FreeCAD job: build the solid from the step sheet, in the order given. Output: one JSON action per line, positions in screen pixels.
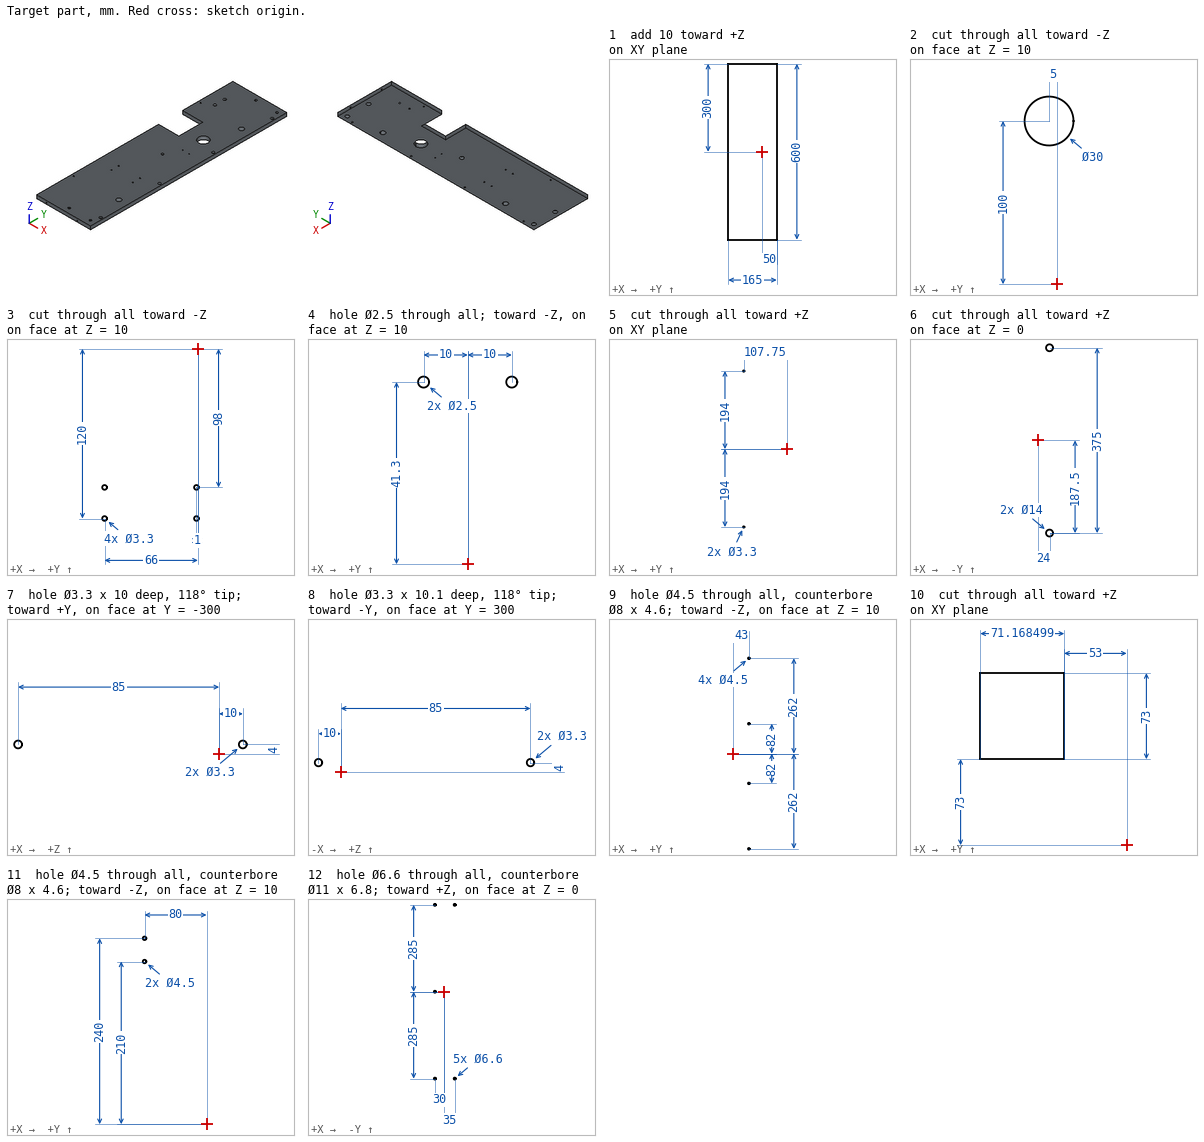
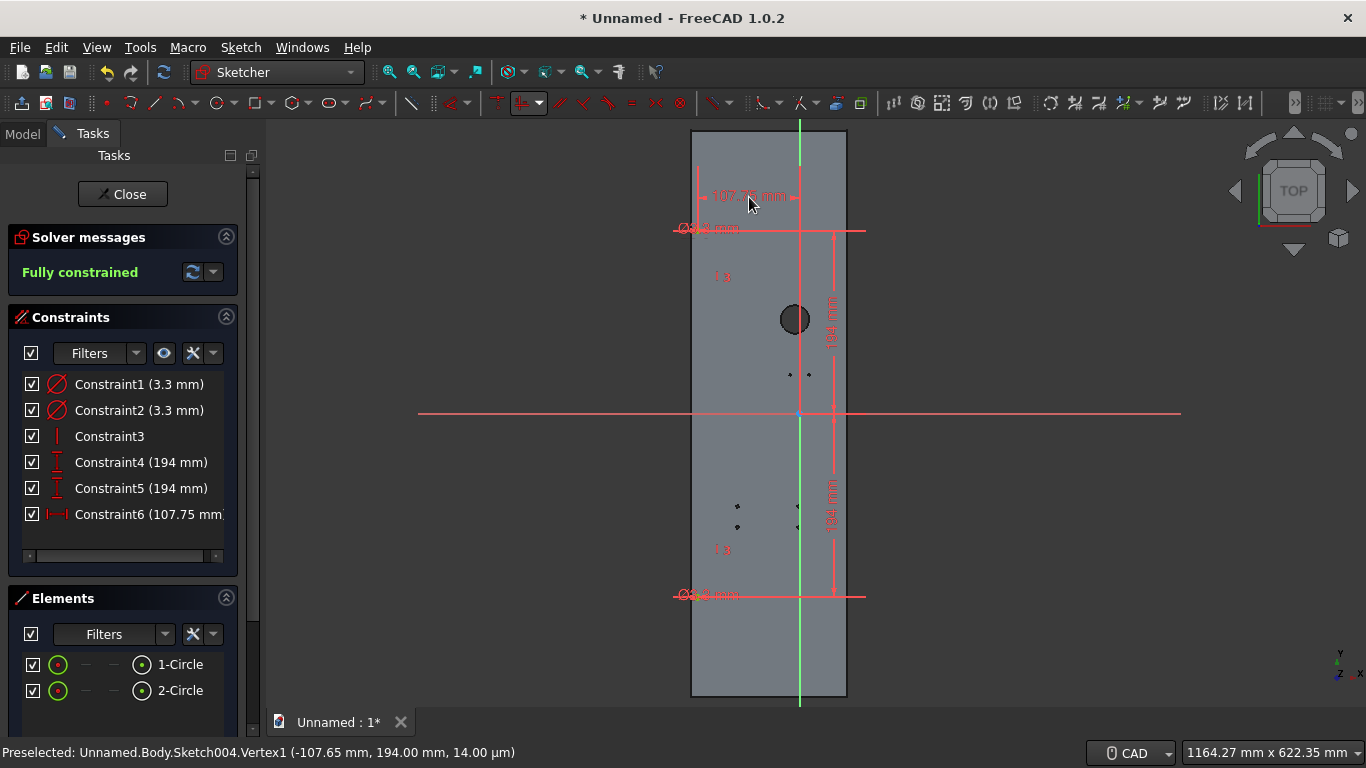
{"action": "left_click", "coordinate": [123, 194]}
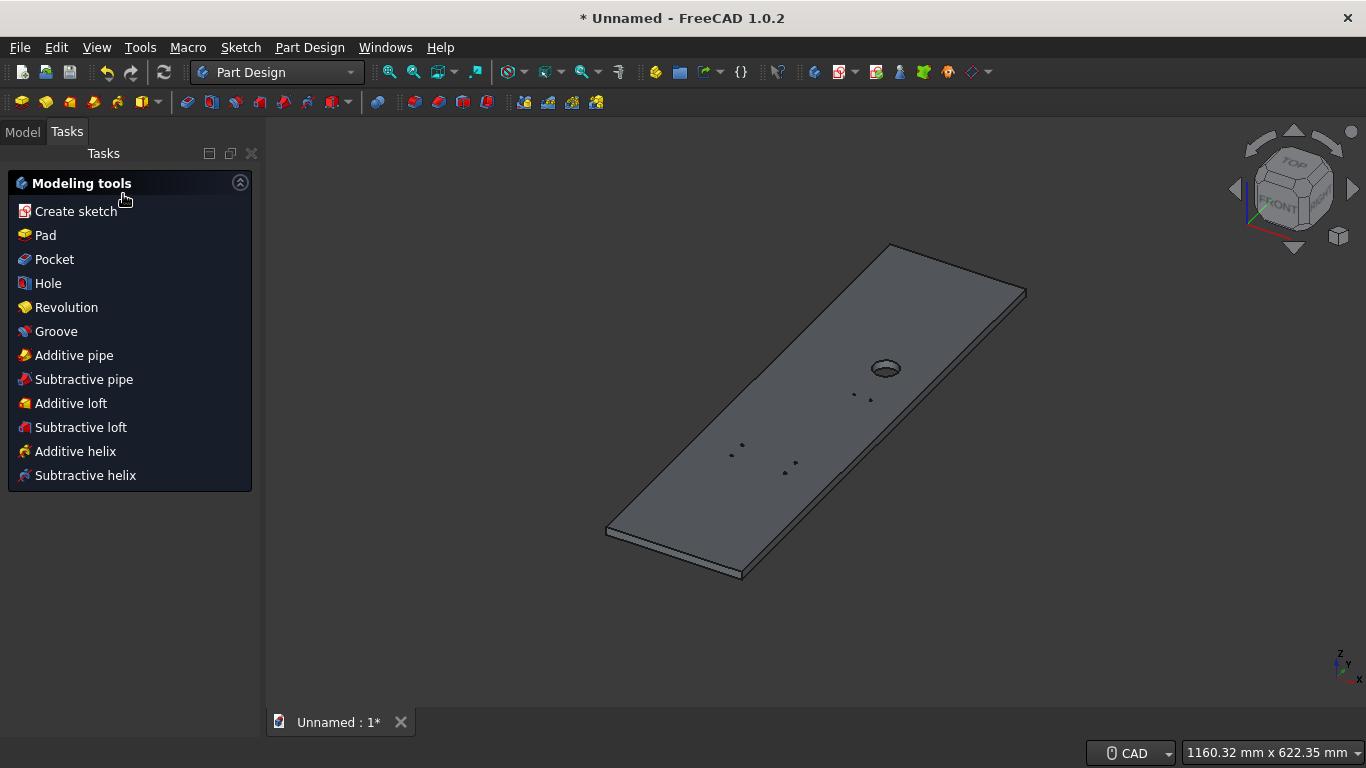
{"action": "left_click", "coordinate": [188, 102]}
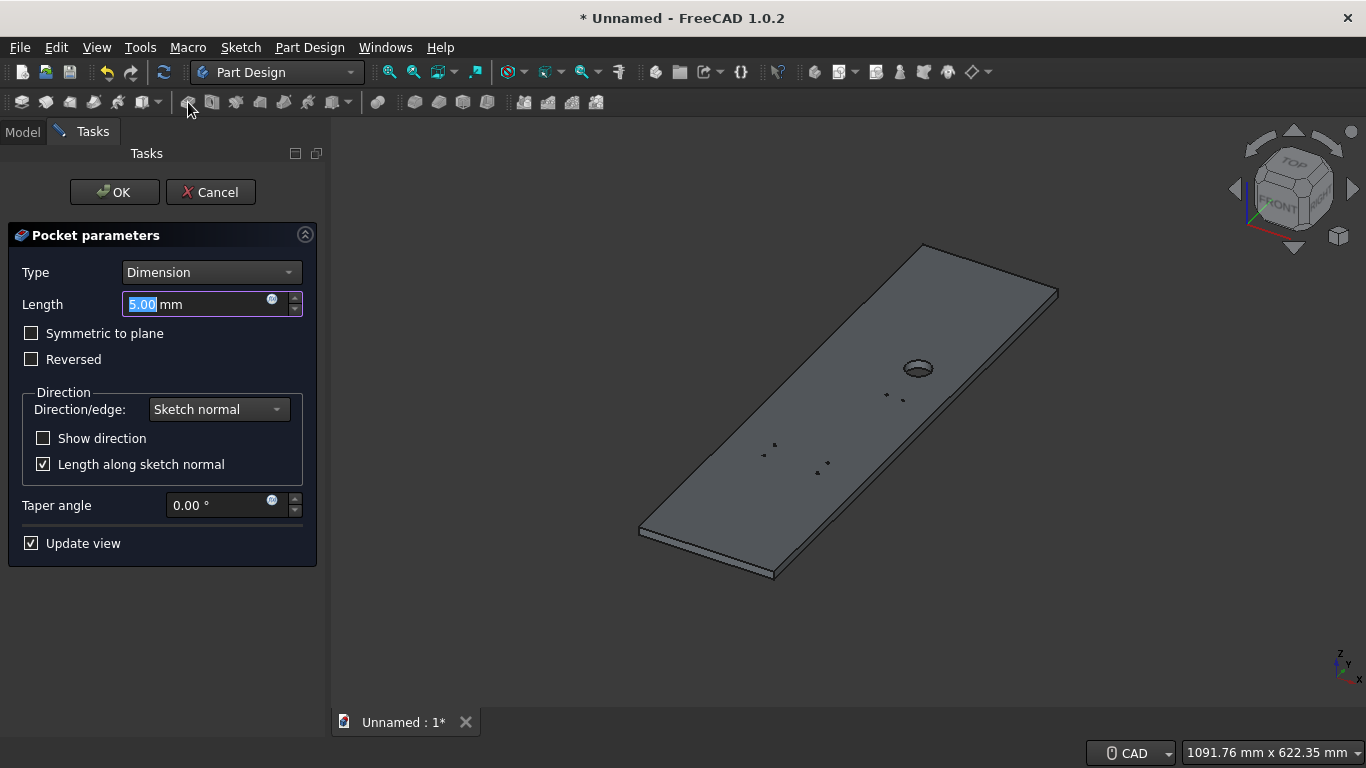
{"action": "left_click", "coordinate": [212, 272]}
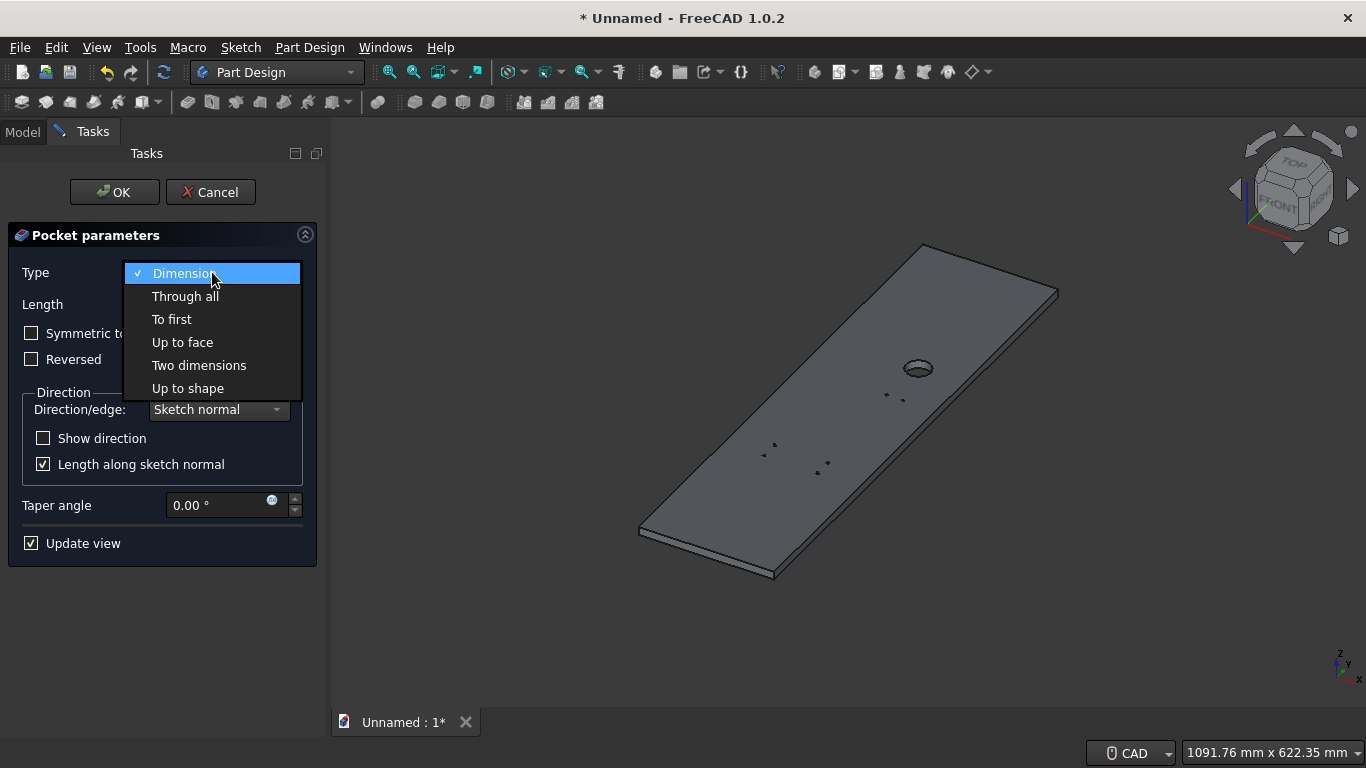
{"action": "left_click", "coordinate": [212, 296]}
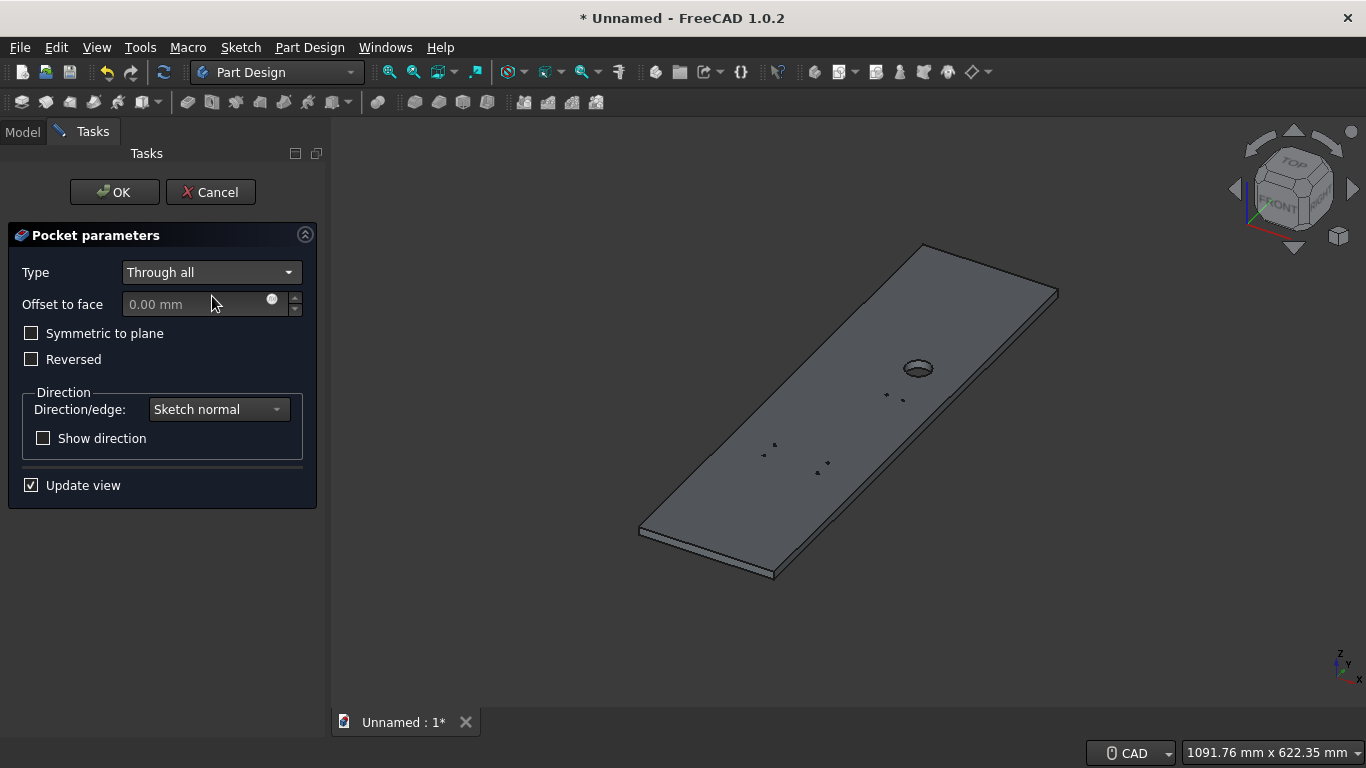
{"action": "left_click", "coordinate": [30, 359]}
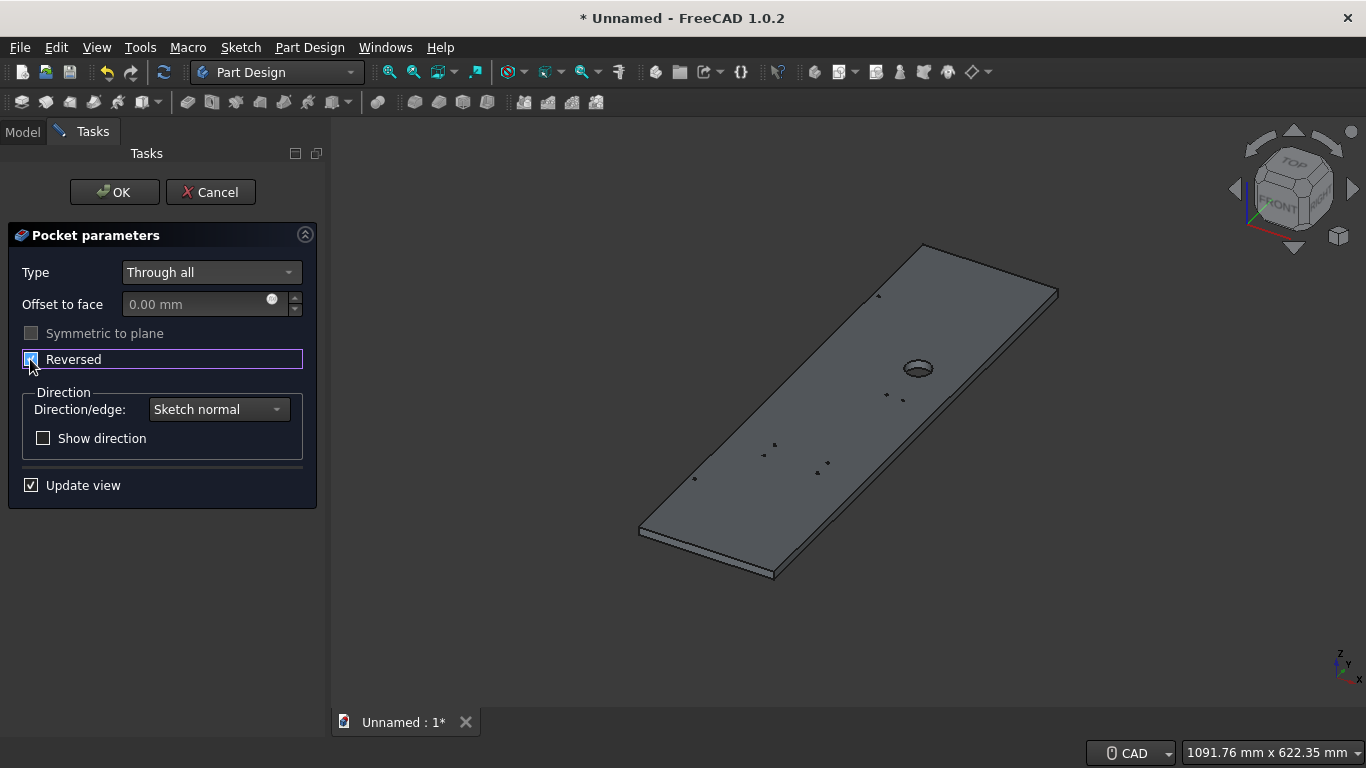
{"action": "left_click", "coordinate": [115, 192]}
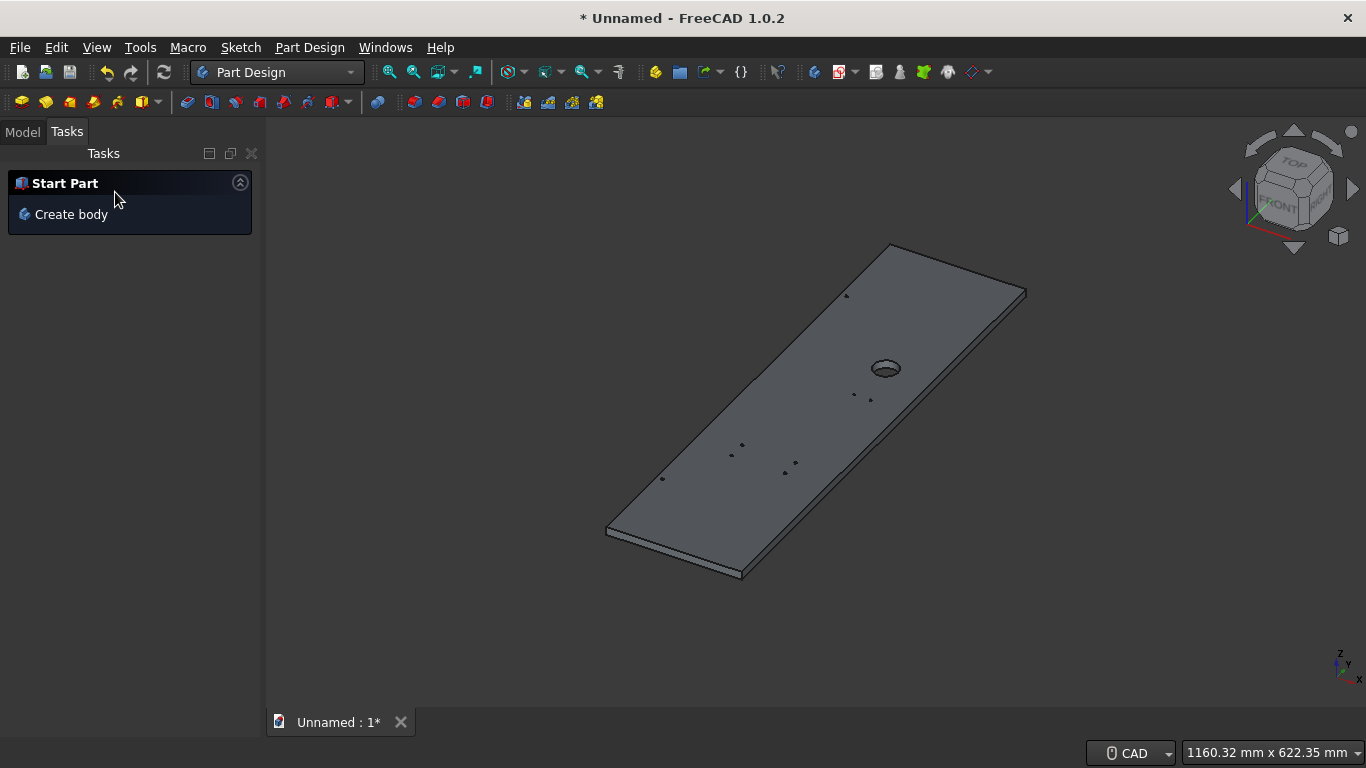
{"action": "key", "text": "5"}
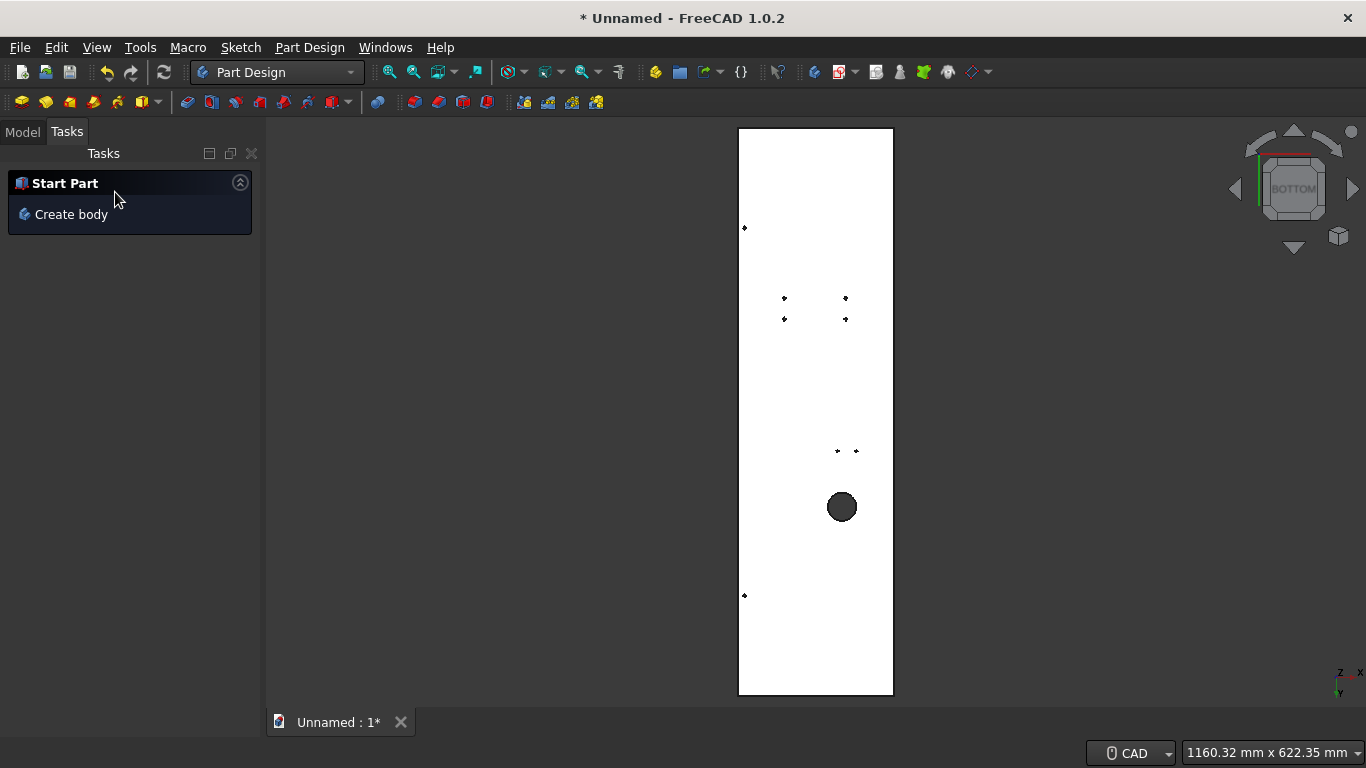
{"action": "left_click", "coordinate": [816, 574]}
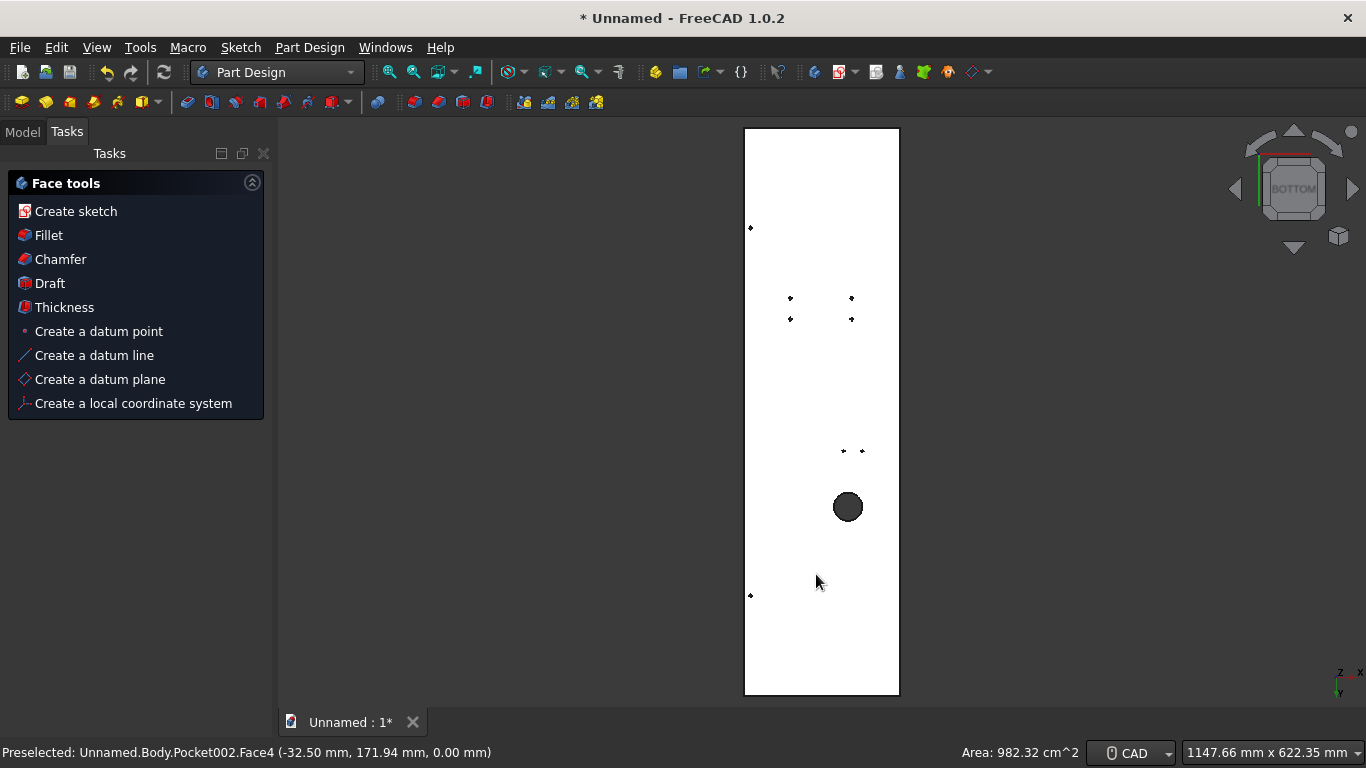
{"action": "left_click", "coordinate": [840, 72]}